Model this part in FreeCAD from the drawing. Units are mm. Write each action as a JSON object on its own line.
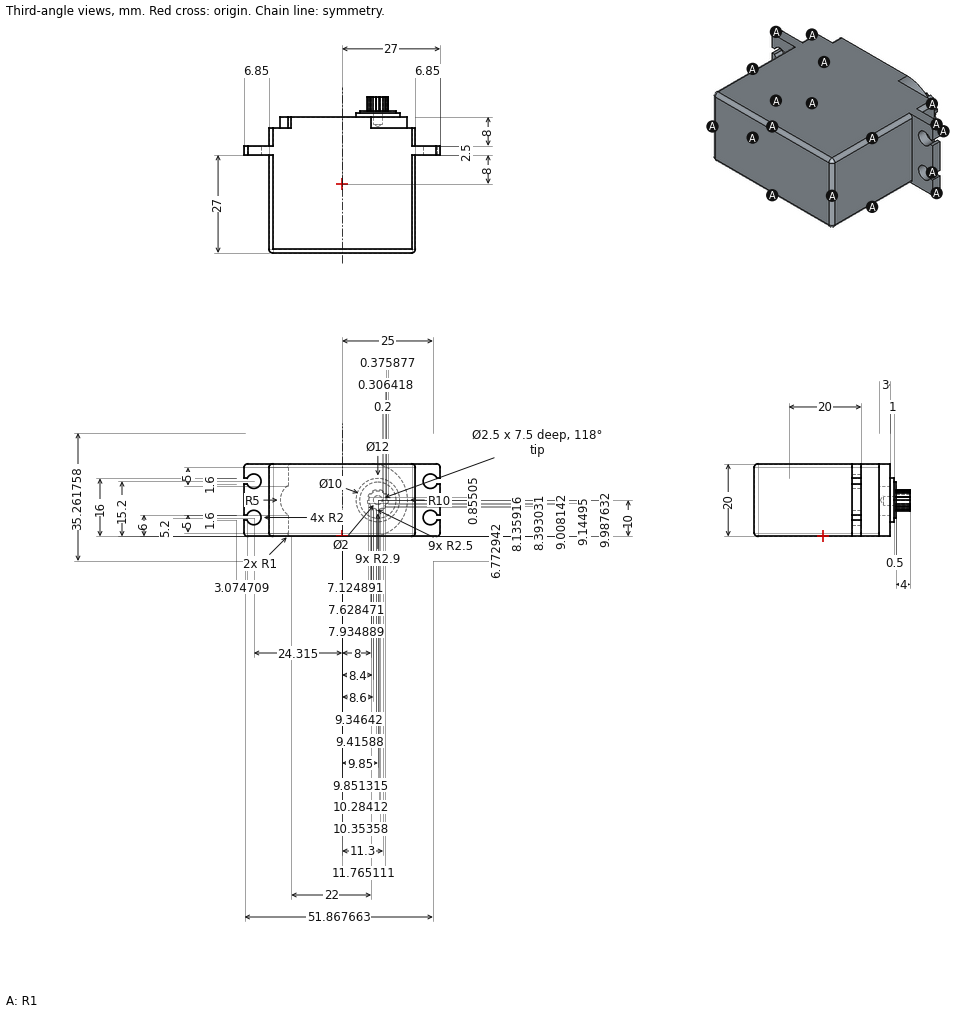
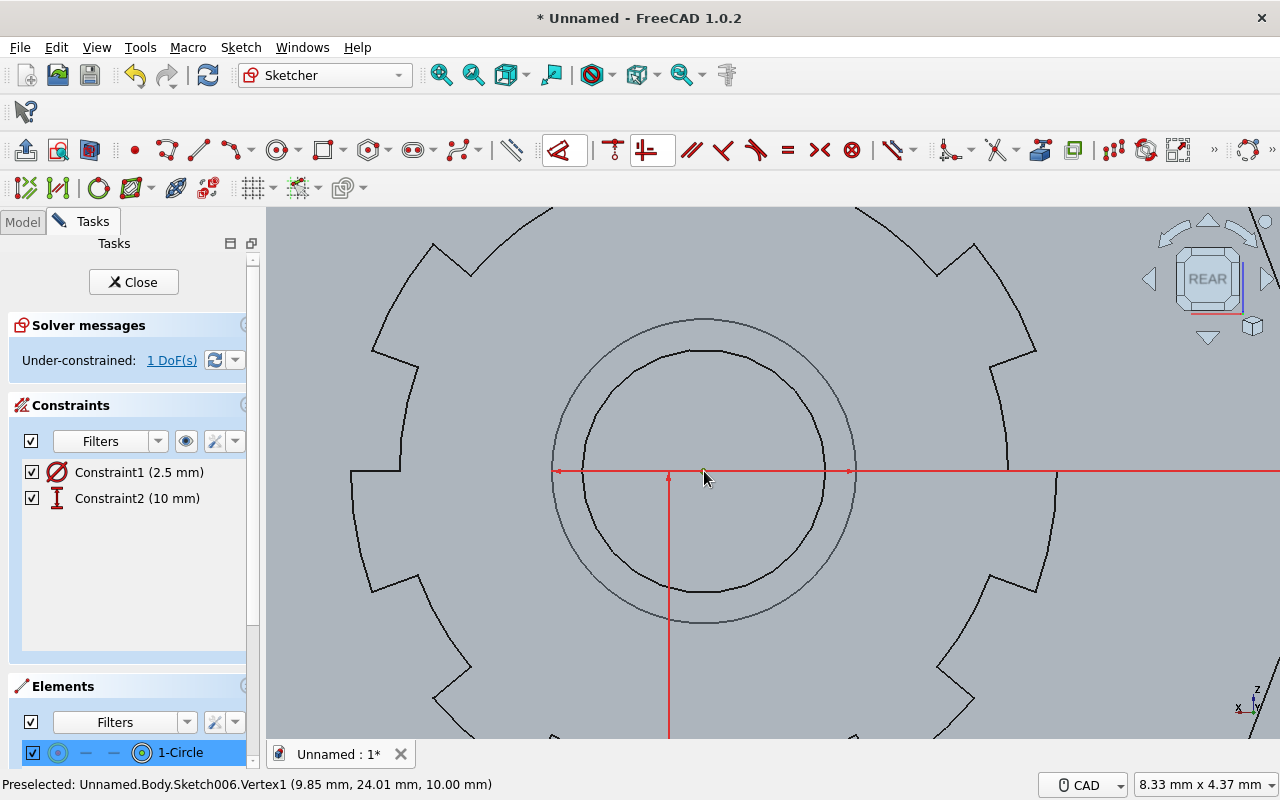
{"action": "key", "text": "l"}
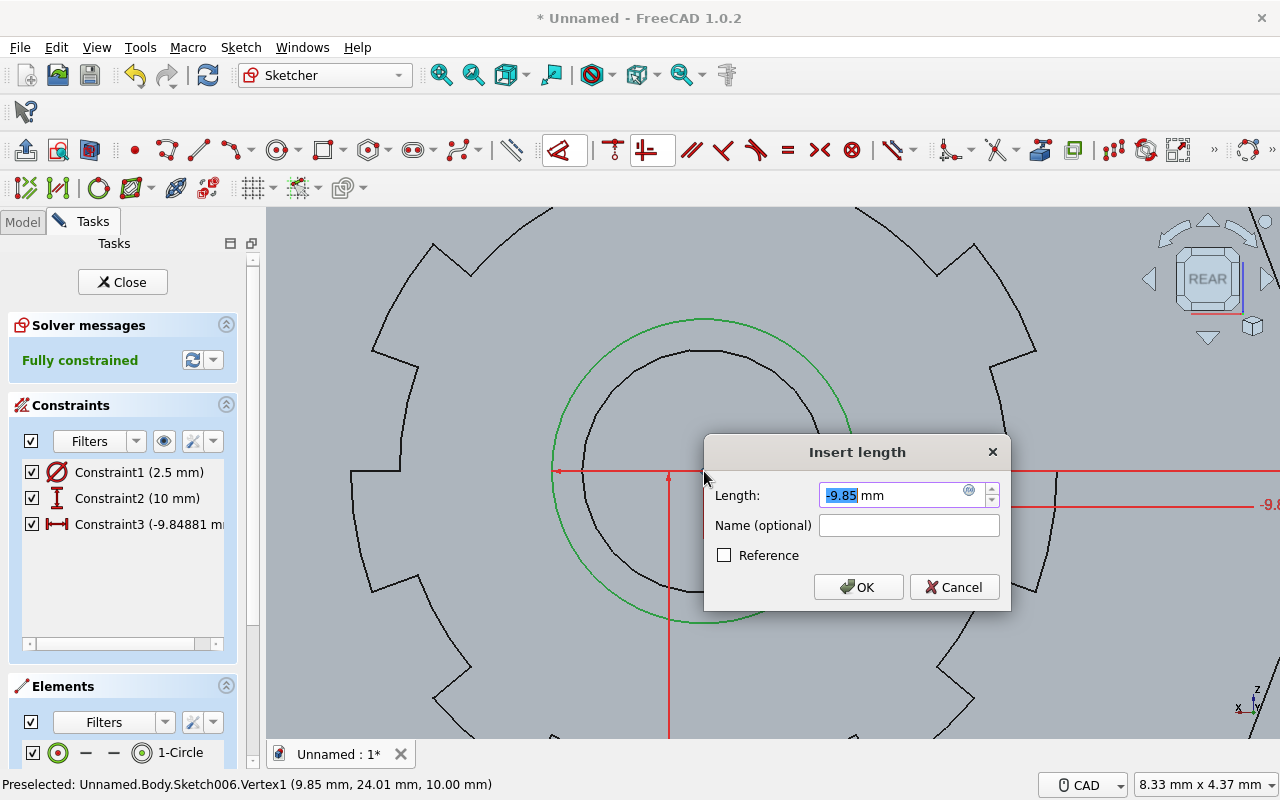
{"action": "type", "text": "-9.85"}
{"action": "key", "text": "Return"}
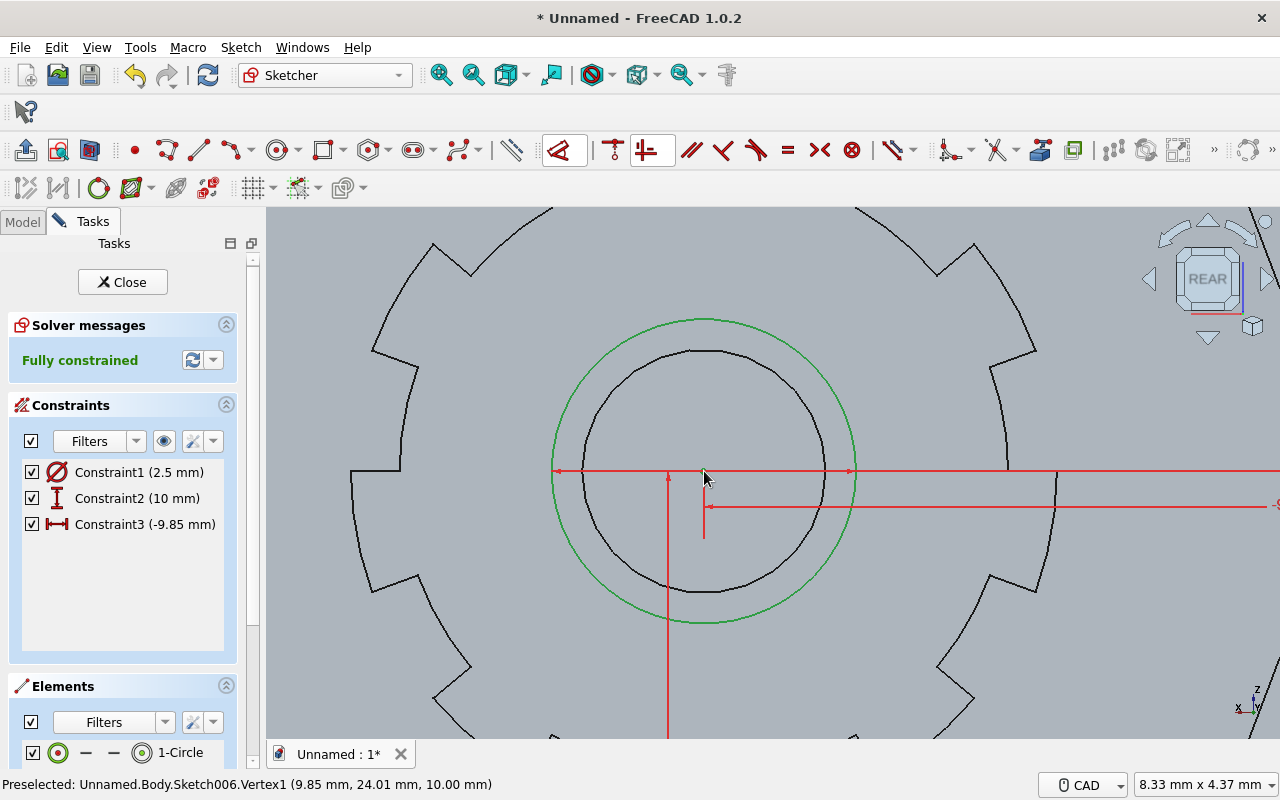
{"action": "left_click", "coordinate": [123, 282]}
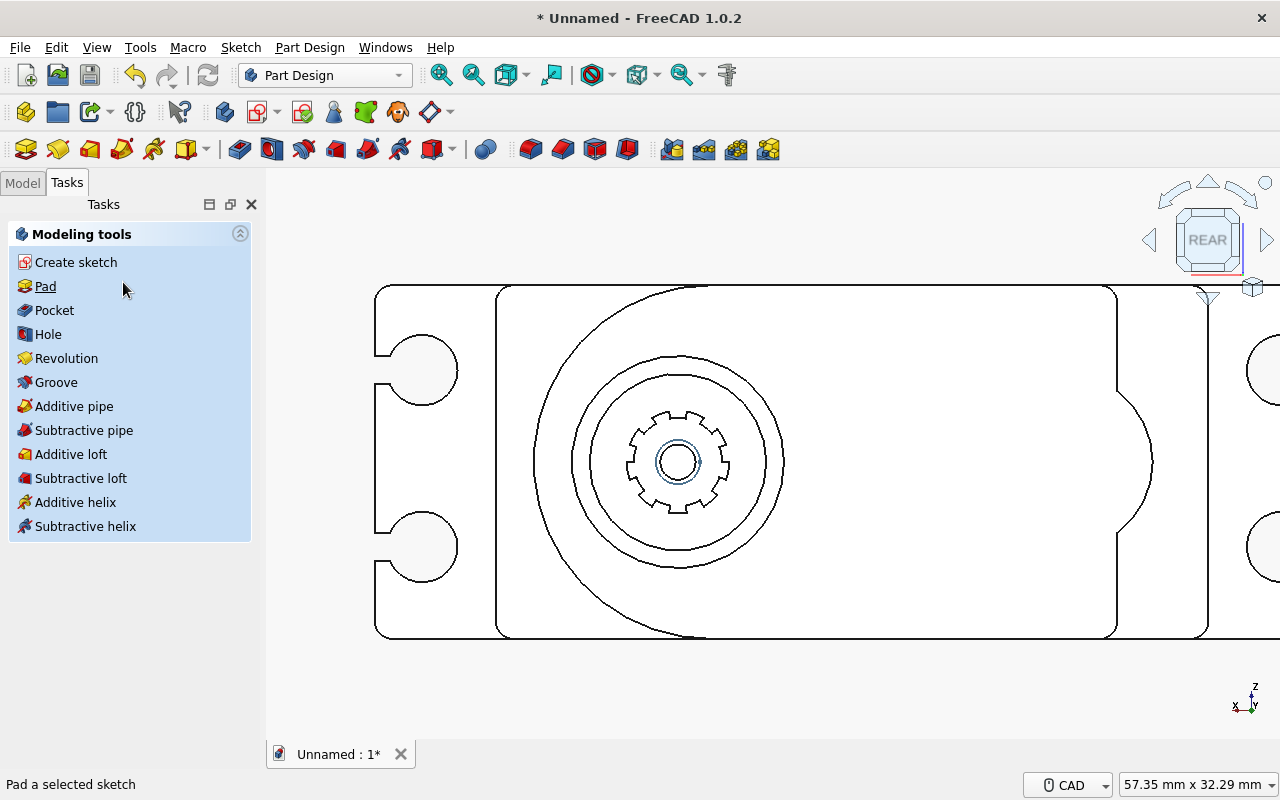
{"action": "left_click", "coordinate": [272, 150]}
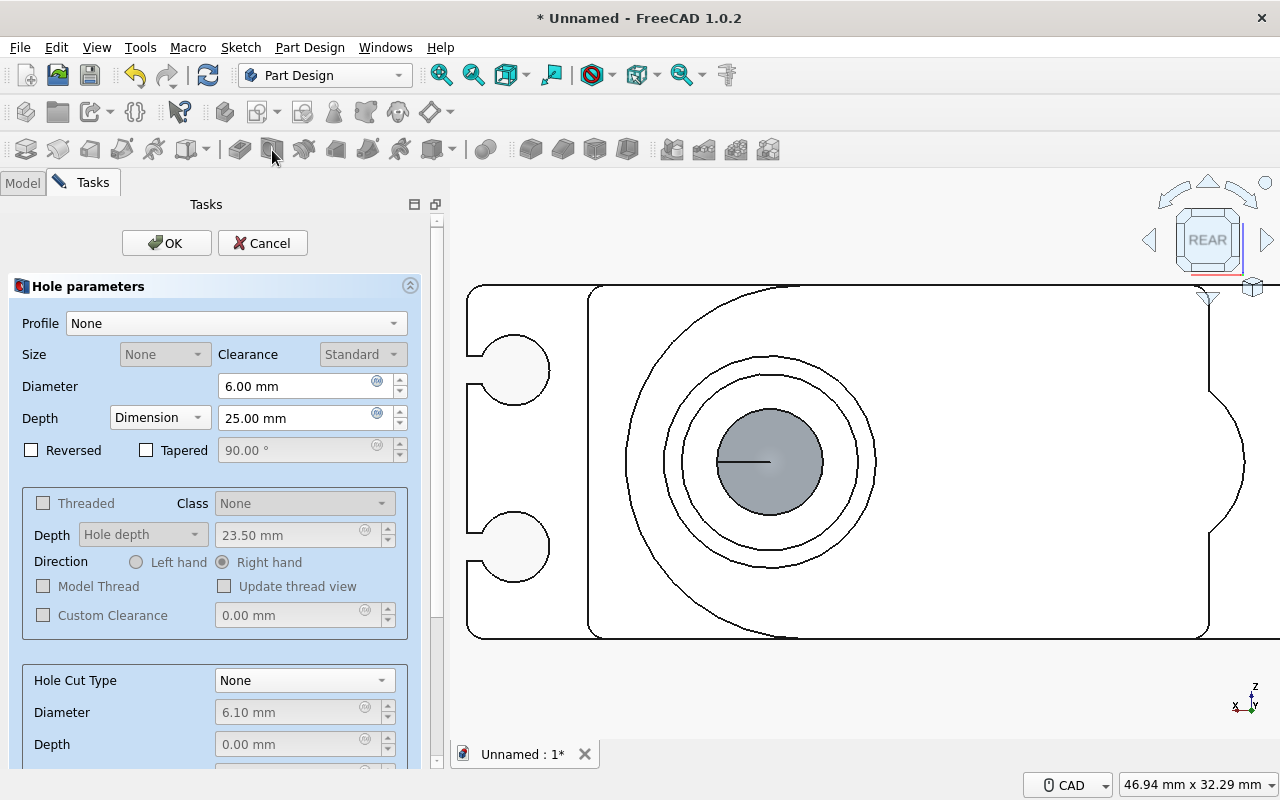
{"action": "triple_click", "coordinate": [305, 386]}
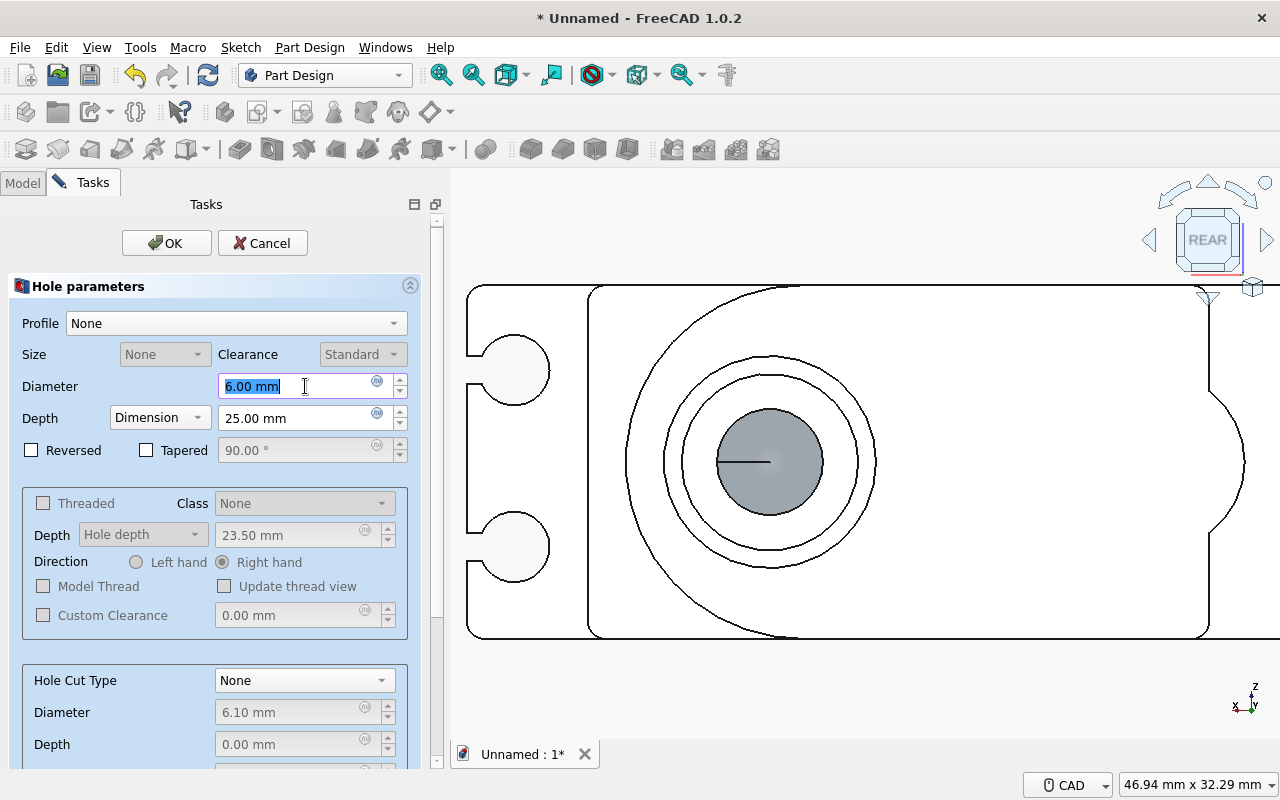
{"action": "type", "text": "2.5"}
{"action": "key", "text": "Tab"}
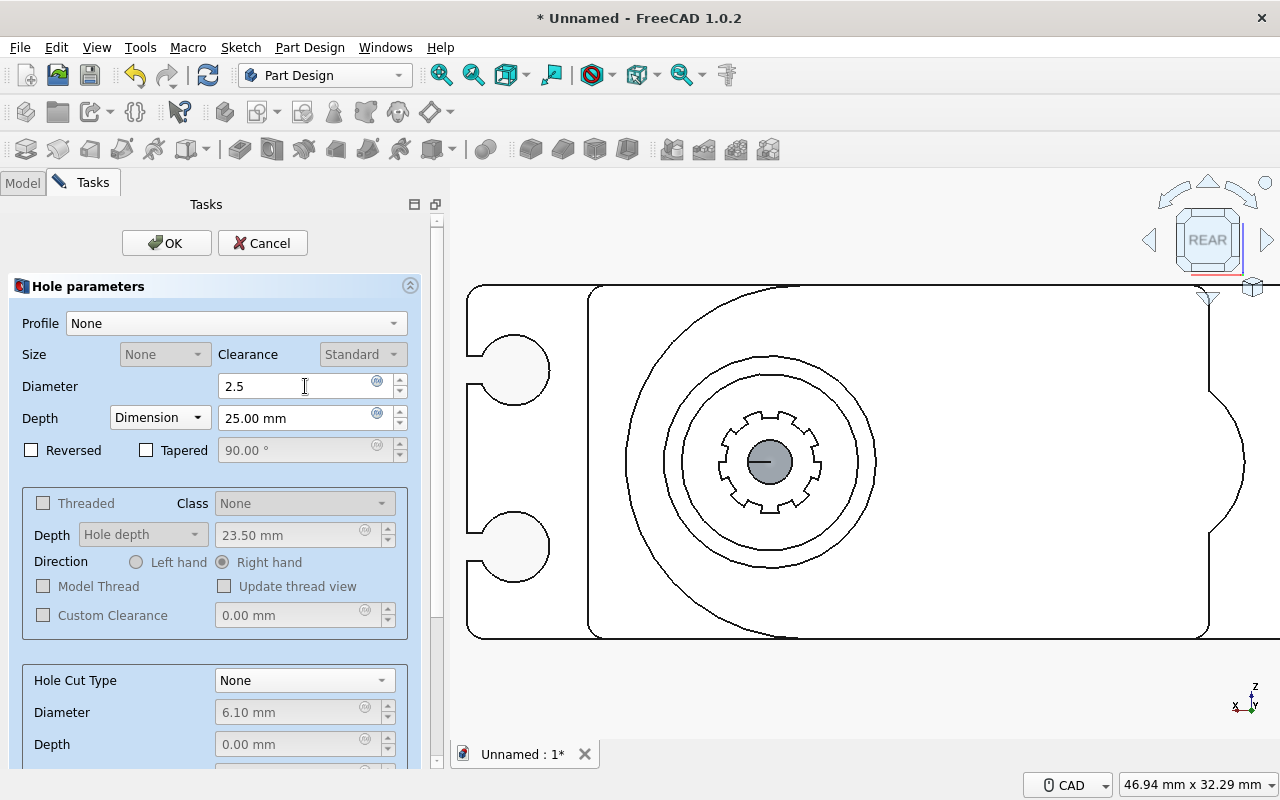
{"action": "triple_click", "coordinate": [305, 418]}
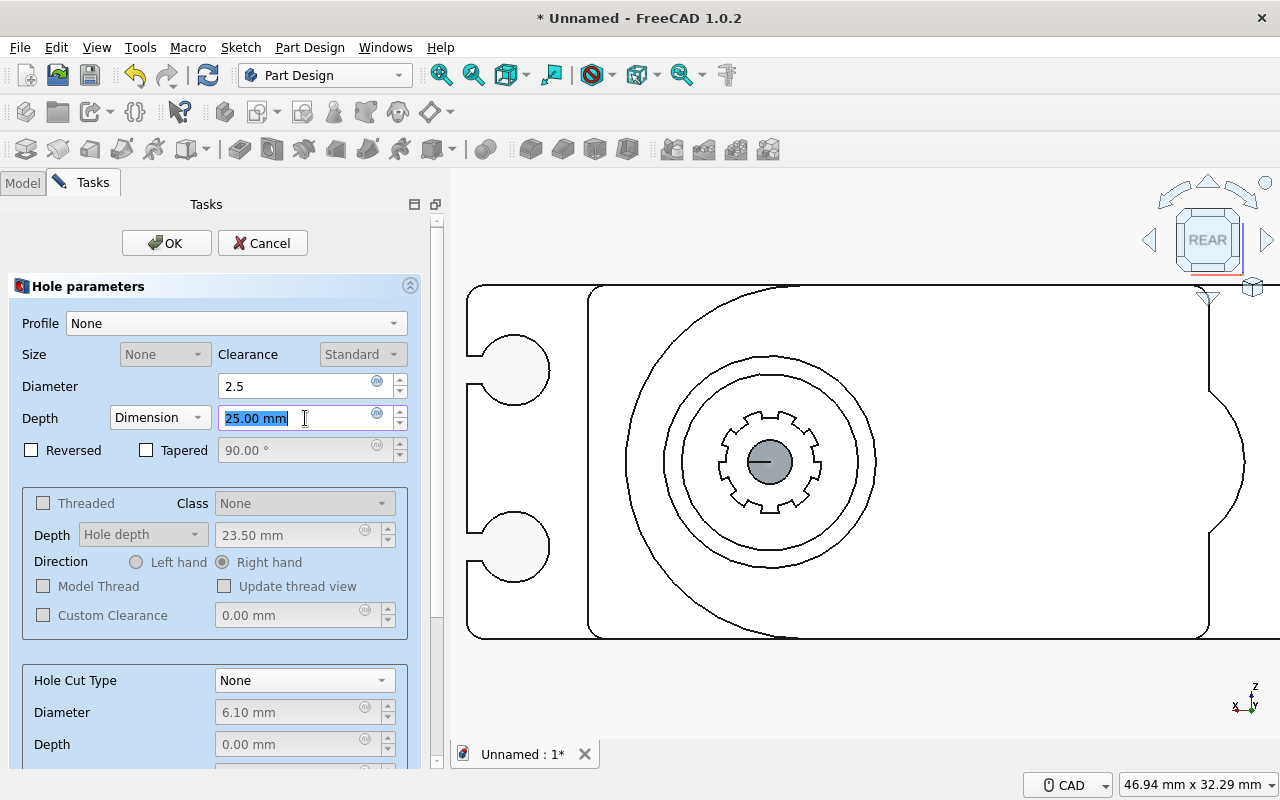
{"action": "type", "text": "7.5"}
{"action": "key", "text": "Tab"}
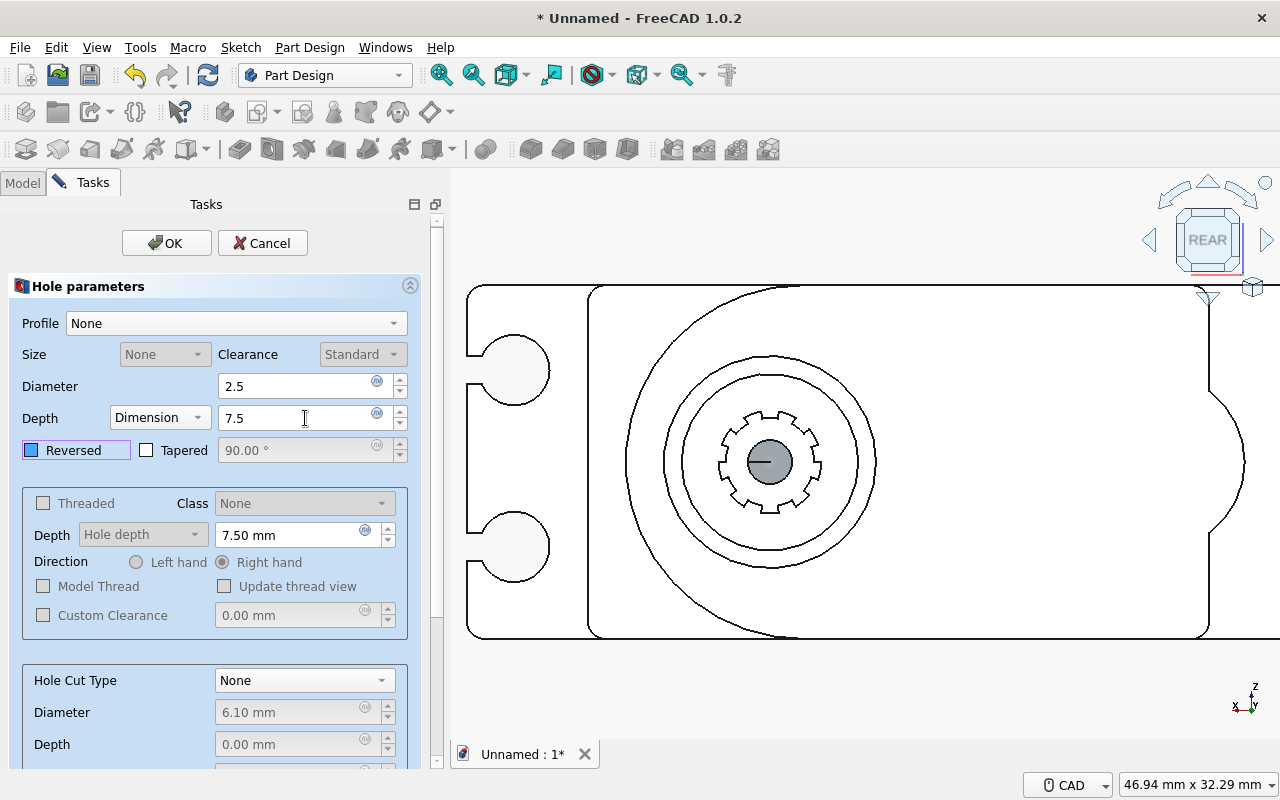
{"action": "left_click", "coordinate": [167, 243]}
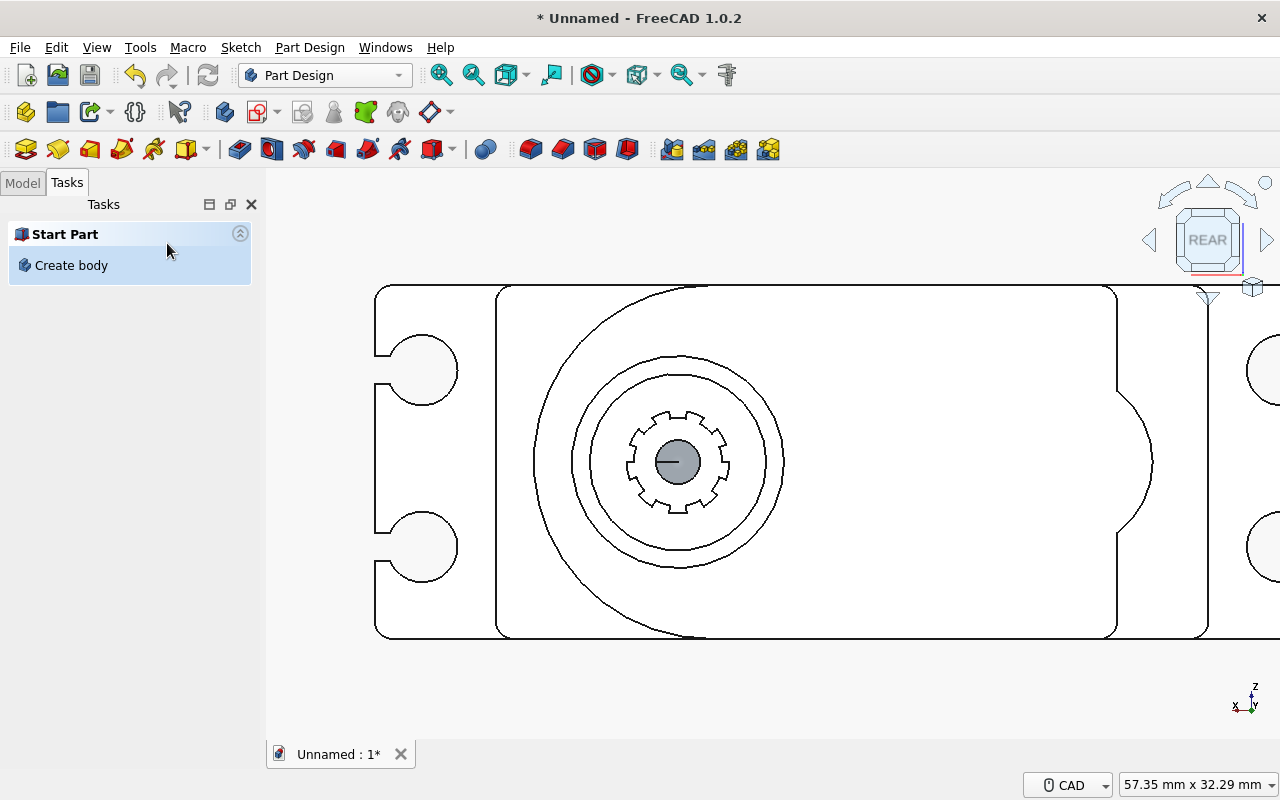
{"action": "key", "text": "0"}